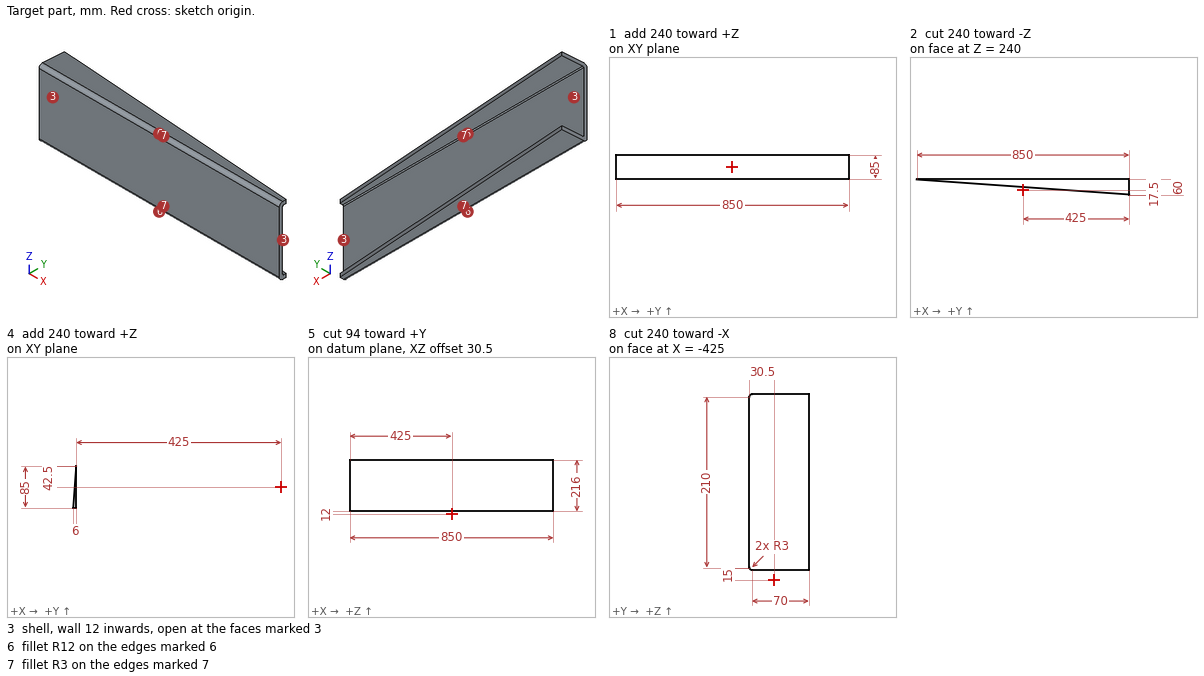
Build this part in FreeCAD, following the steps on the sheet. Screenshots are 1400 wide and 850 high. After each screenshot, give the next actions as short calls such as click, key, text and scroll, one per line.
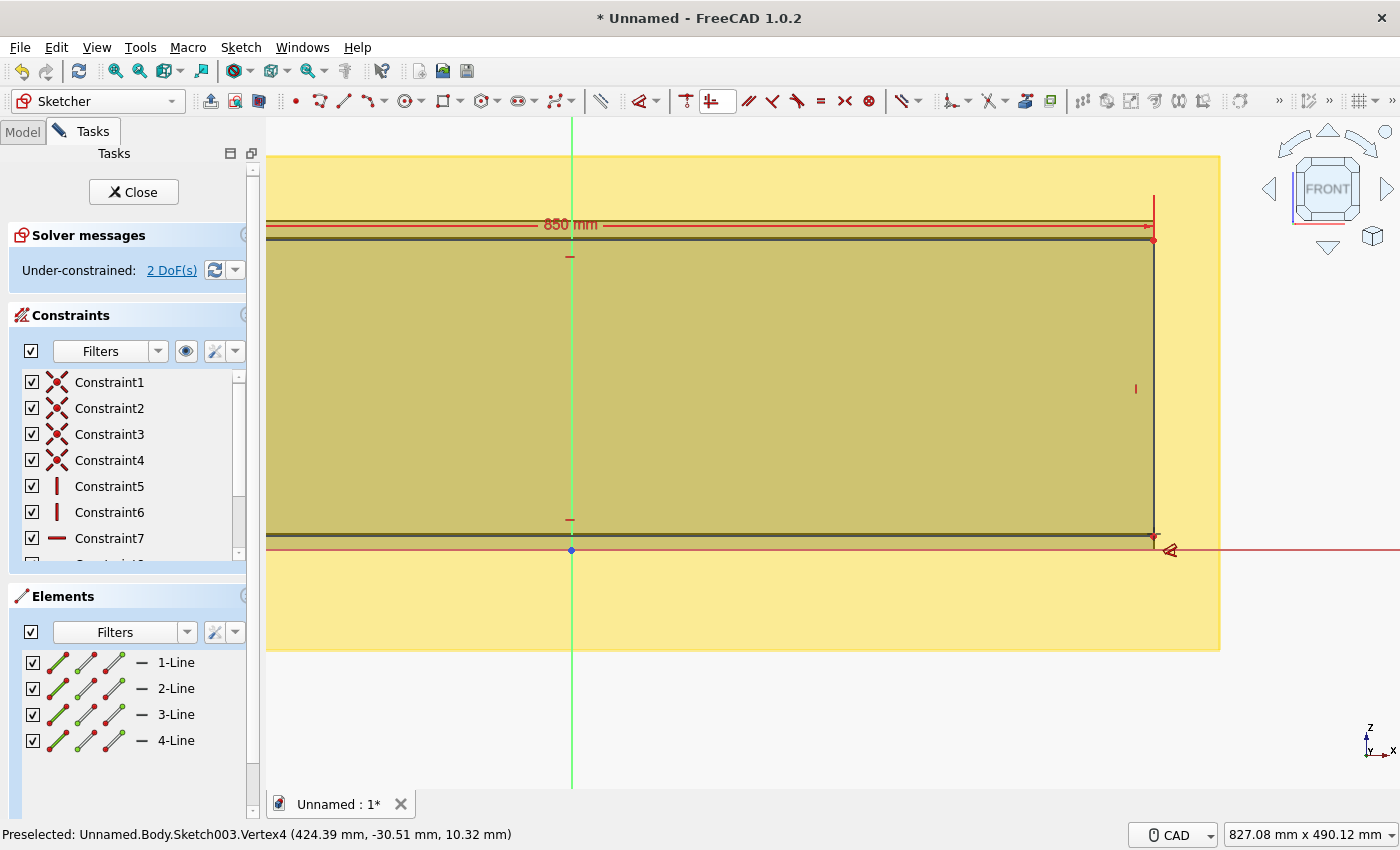
scroll(999, 525, down, 3)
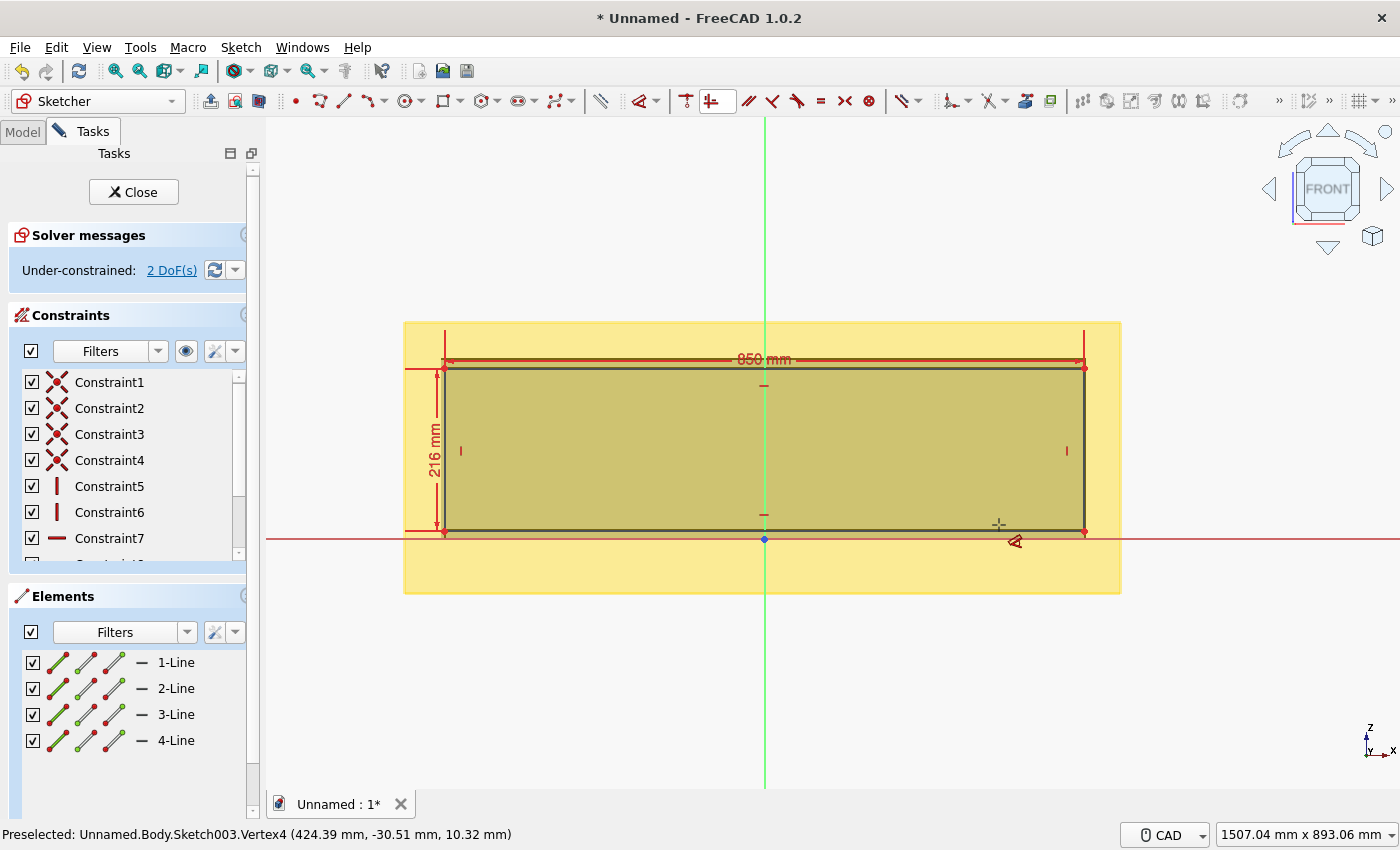
scroll(445, 531, up, 8)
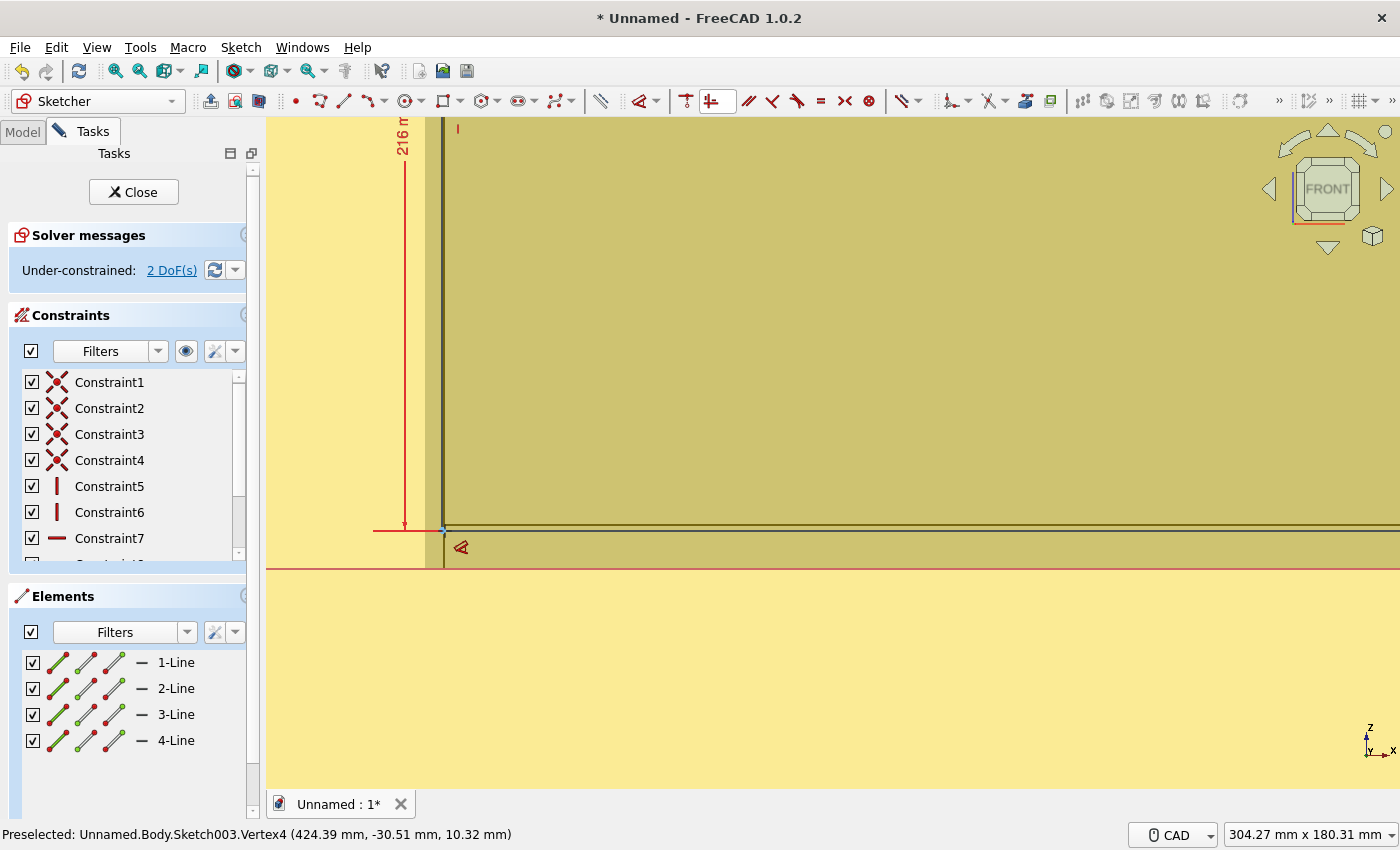
click(442, 531)
click(408, 550)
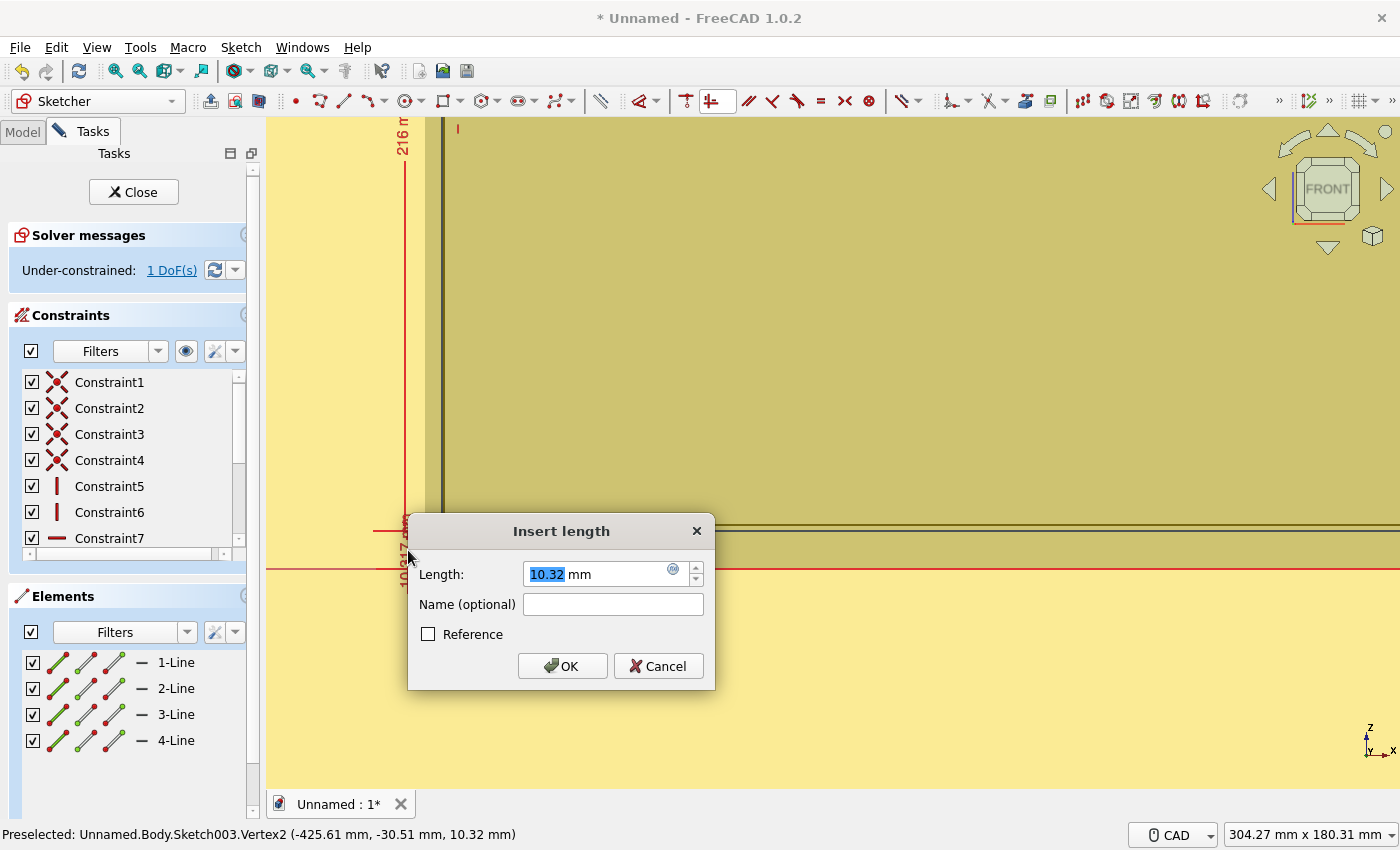
text(12)
key(Return)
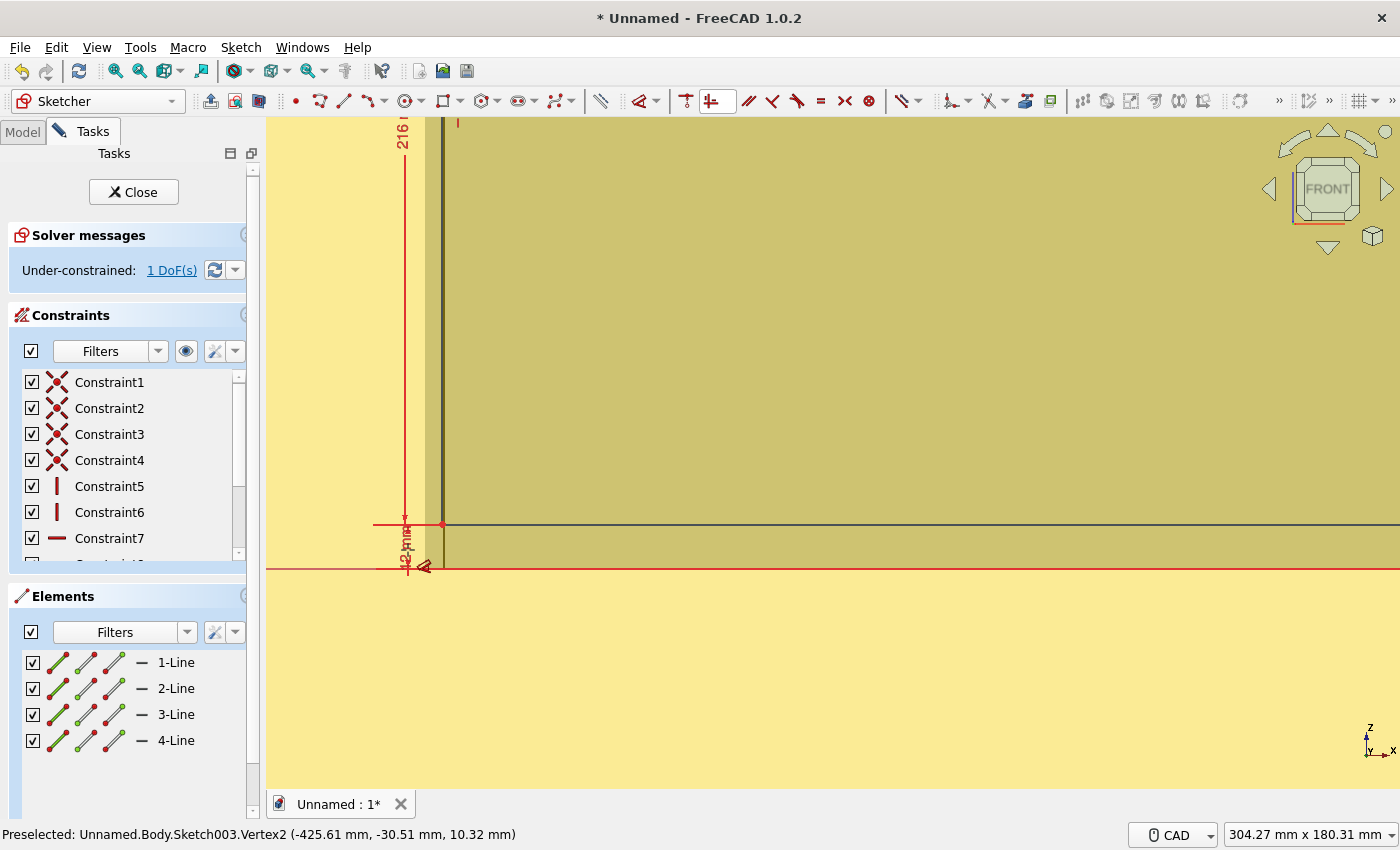
scroll(445, 531, down, 8)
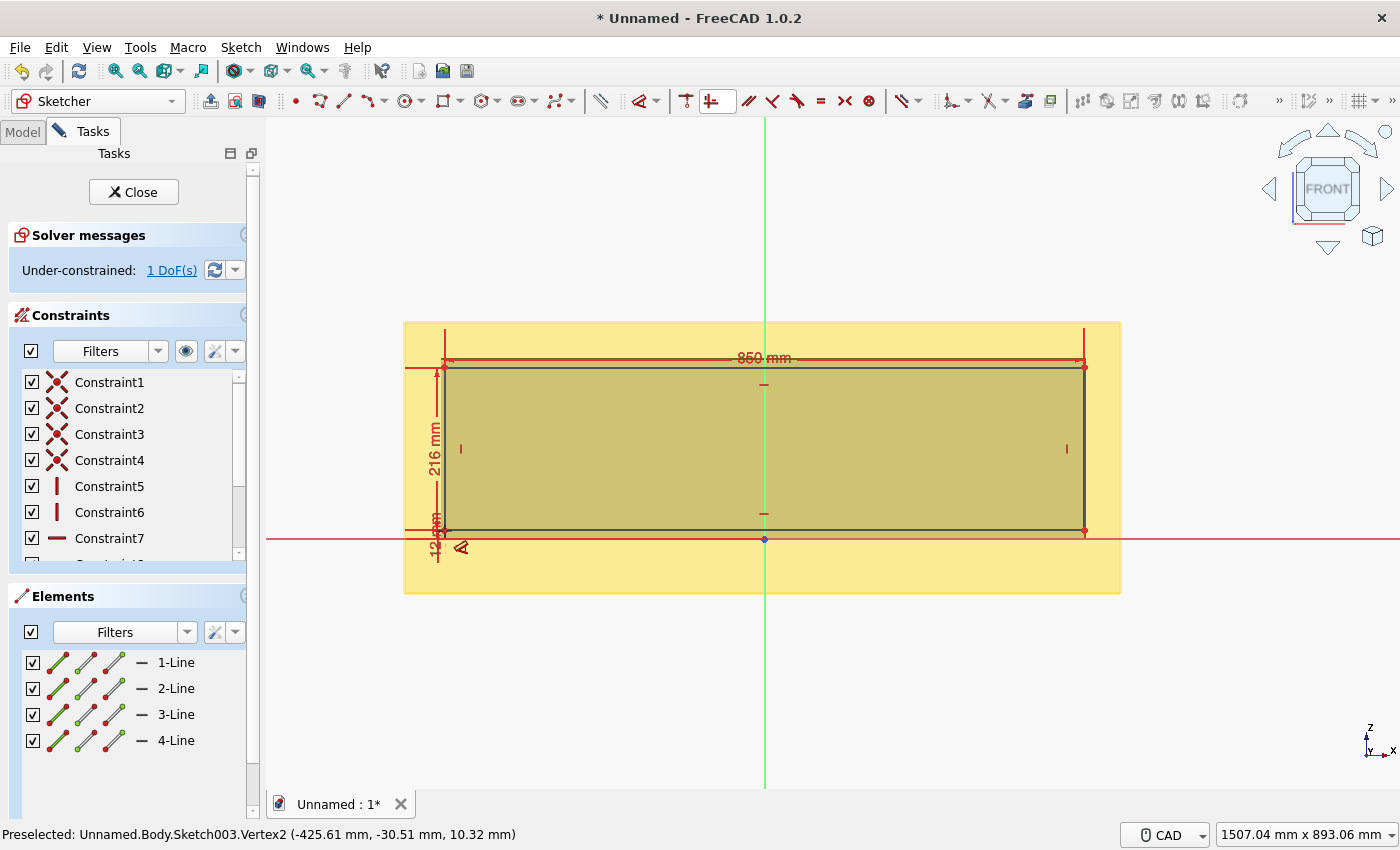
click(445, 368)
click(605, 573)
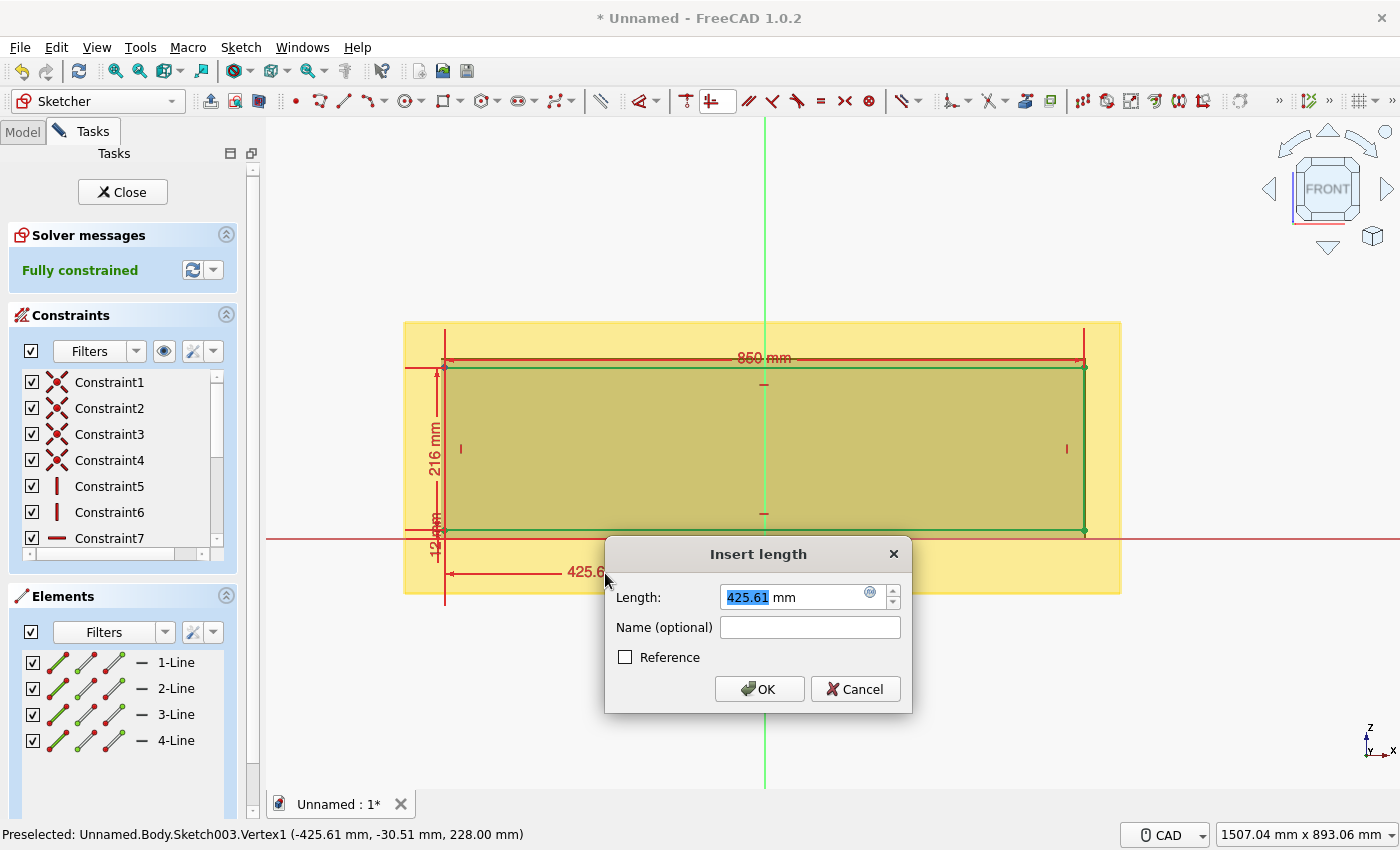
text(425)
key(Return)
key(Escape)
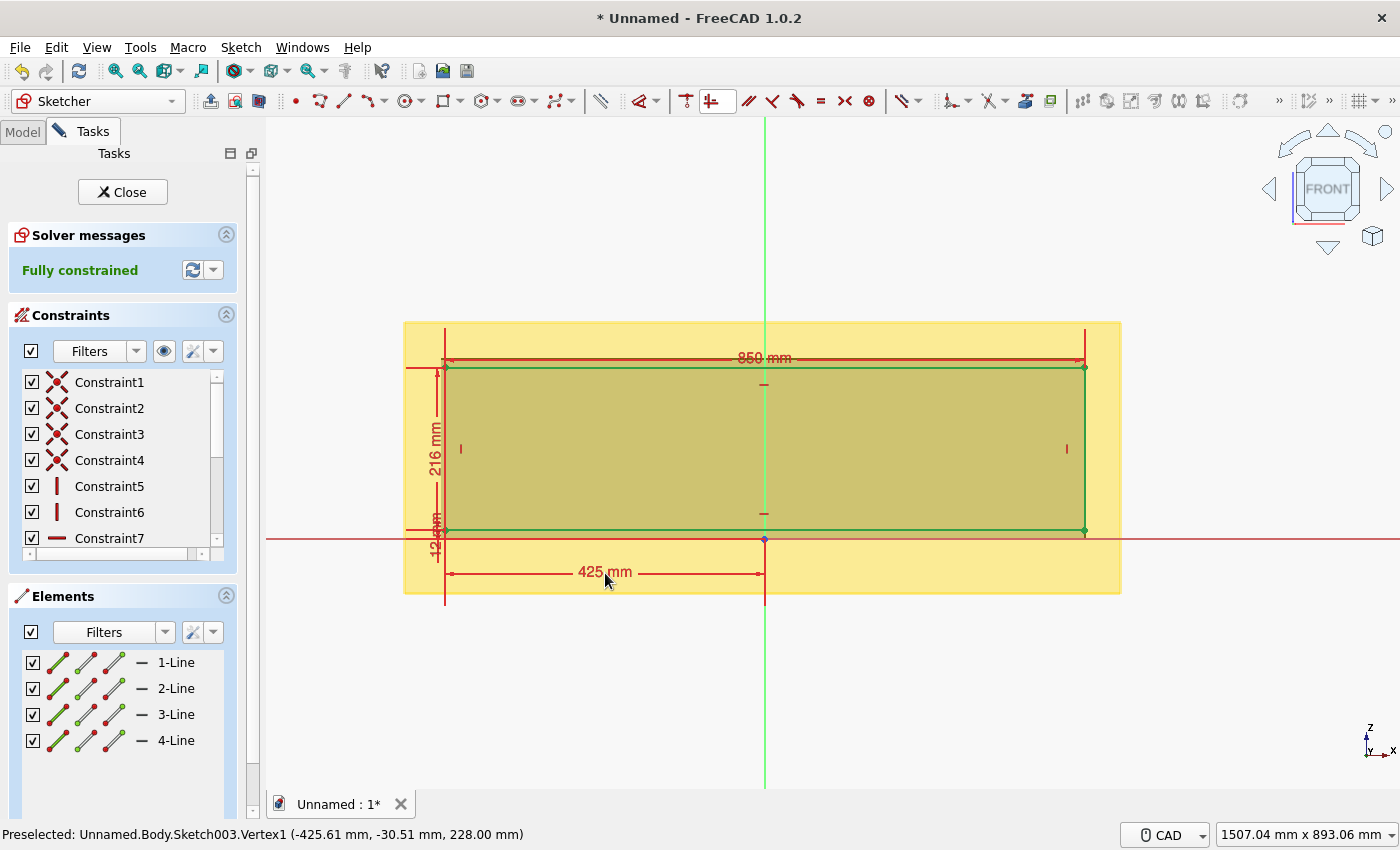
click(123, 192)